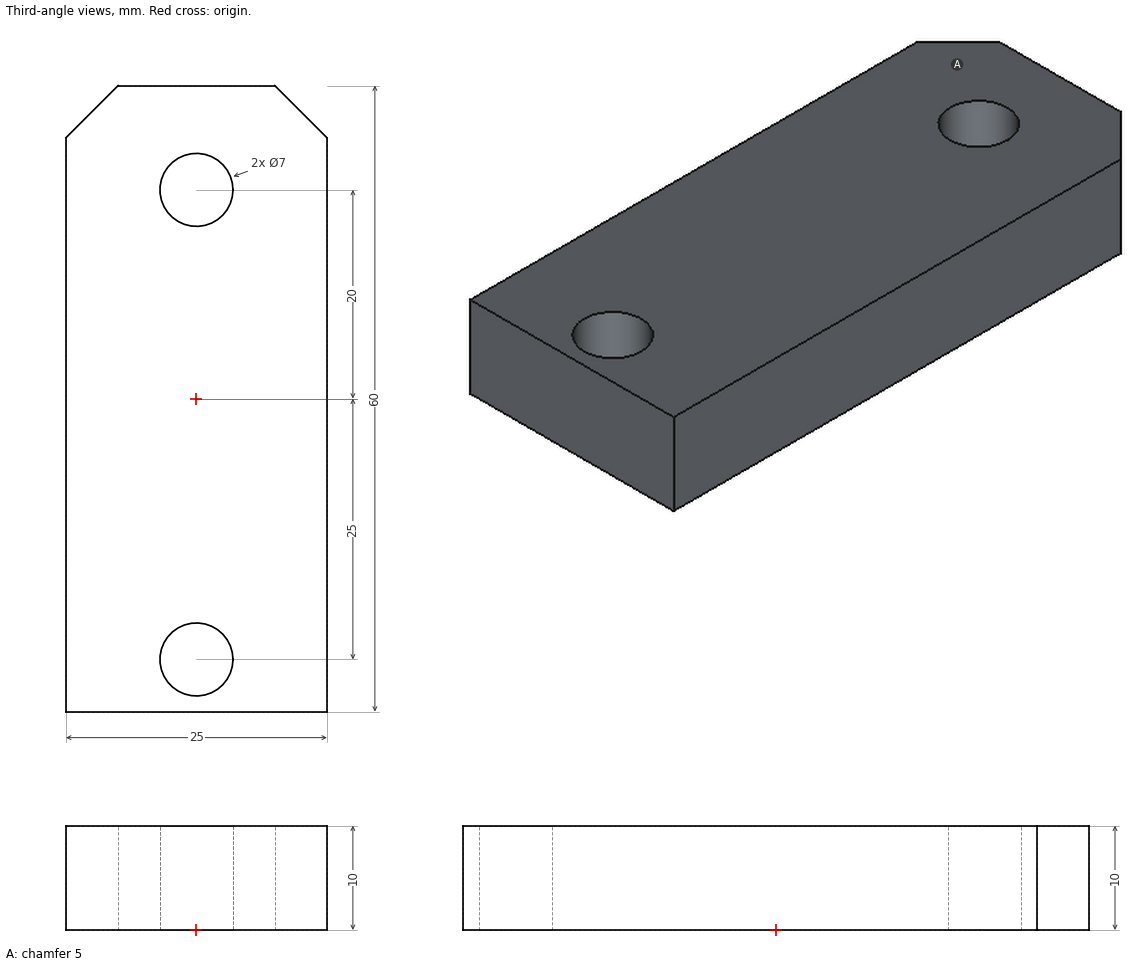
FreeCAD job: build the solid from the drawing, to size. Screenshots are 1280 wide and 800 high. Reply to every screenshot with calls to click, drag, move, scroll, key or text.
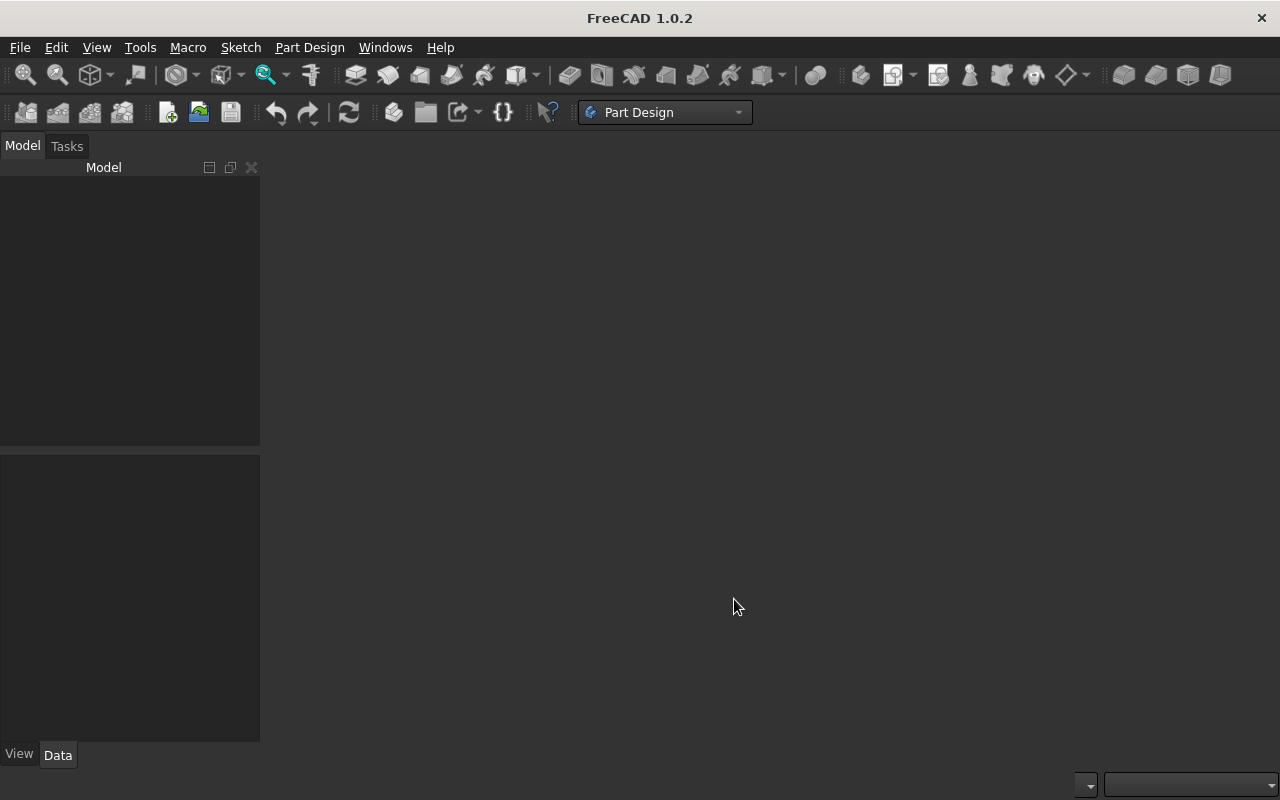
click(168, 112)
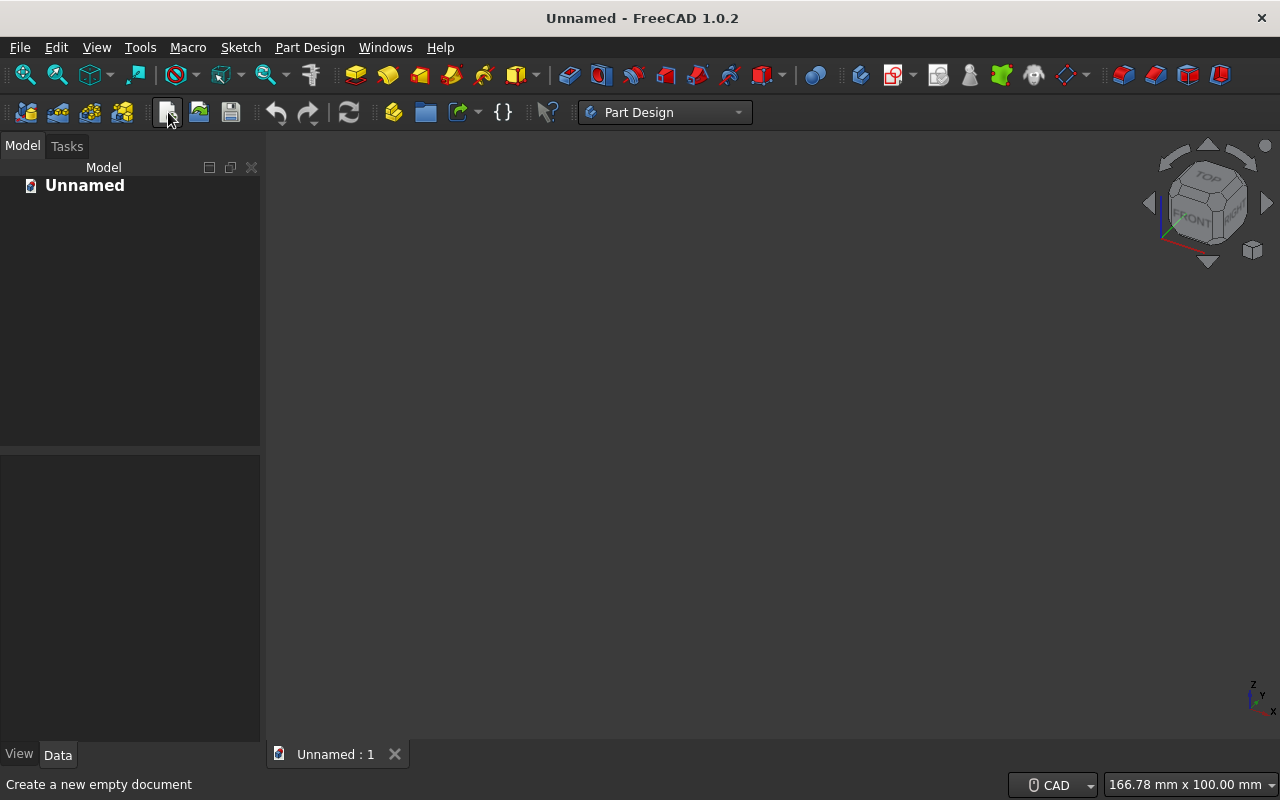
click(894, 76)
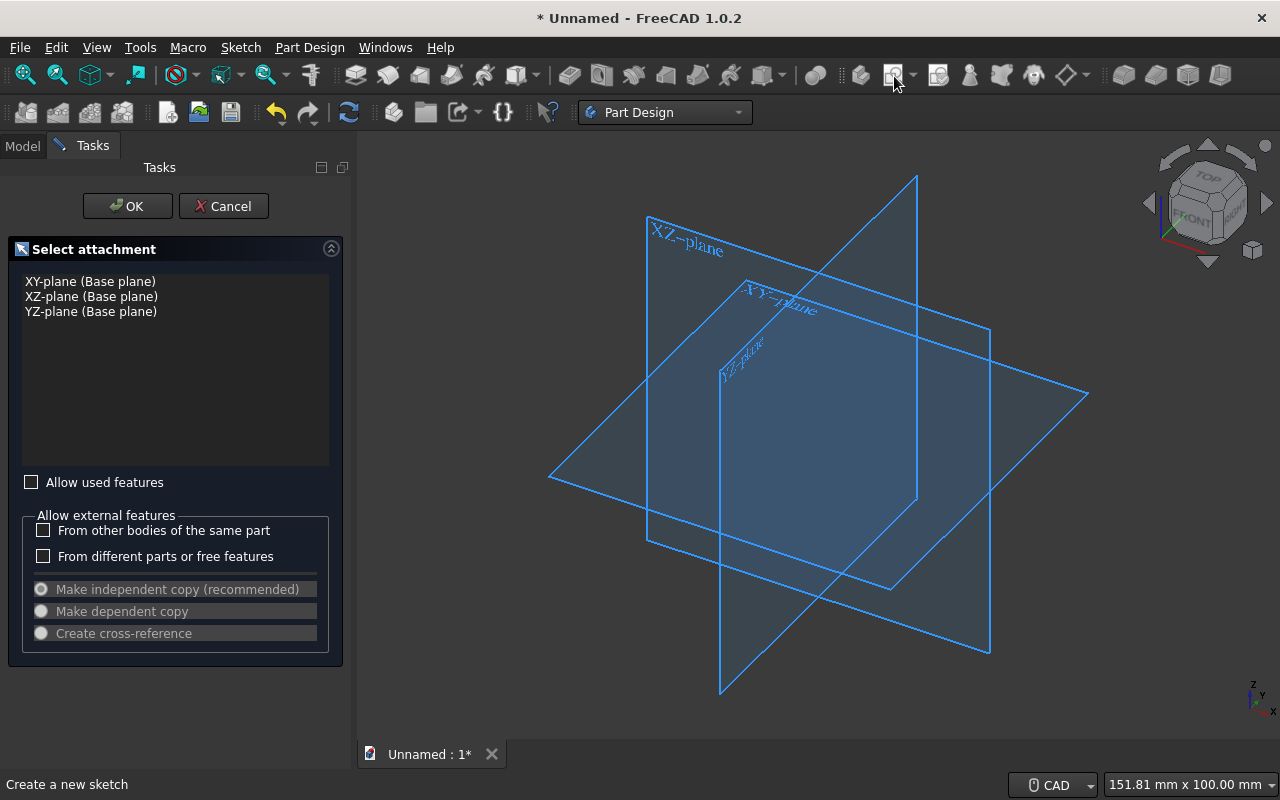
click(82, 282)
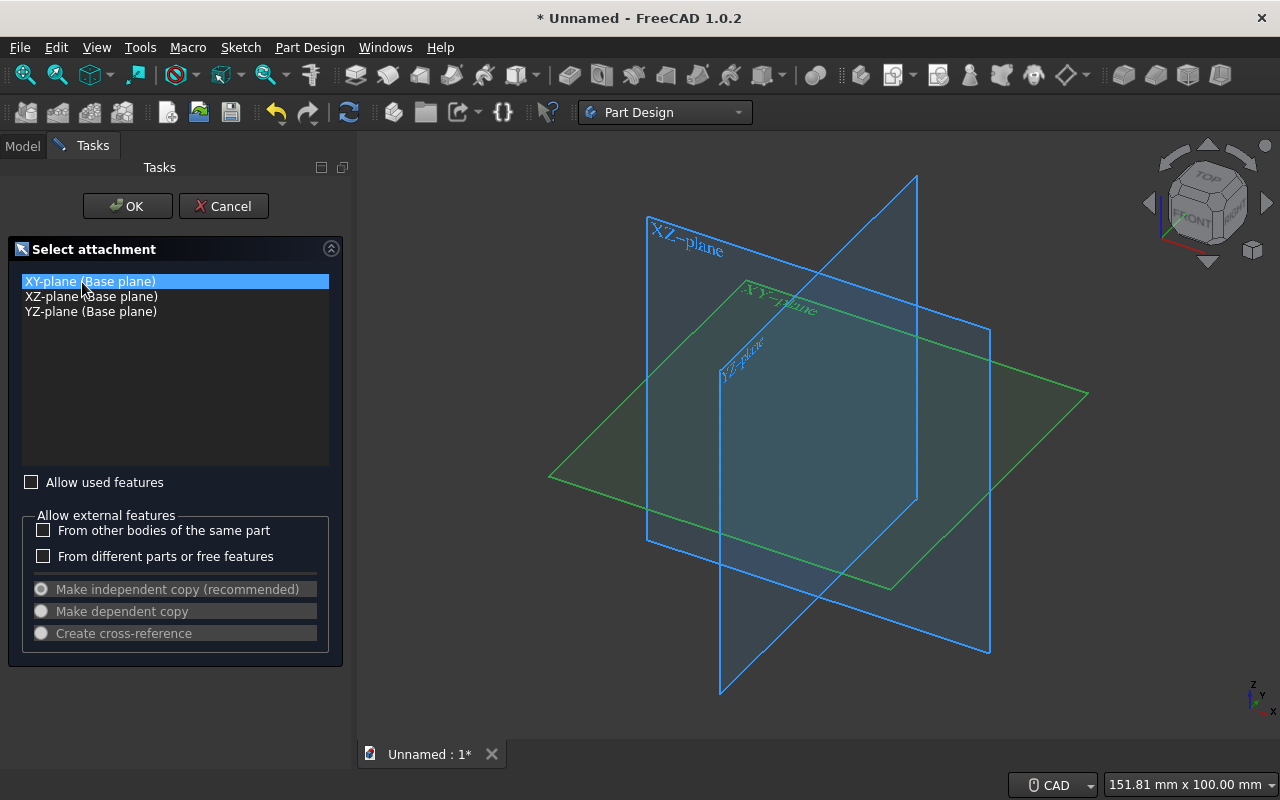
click(128, 206)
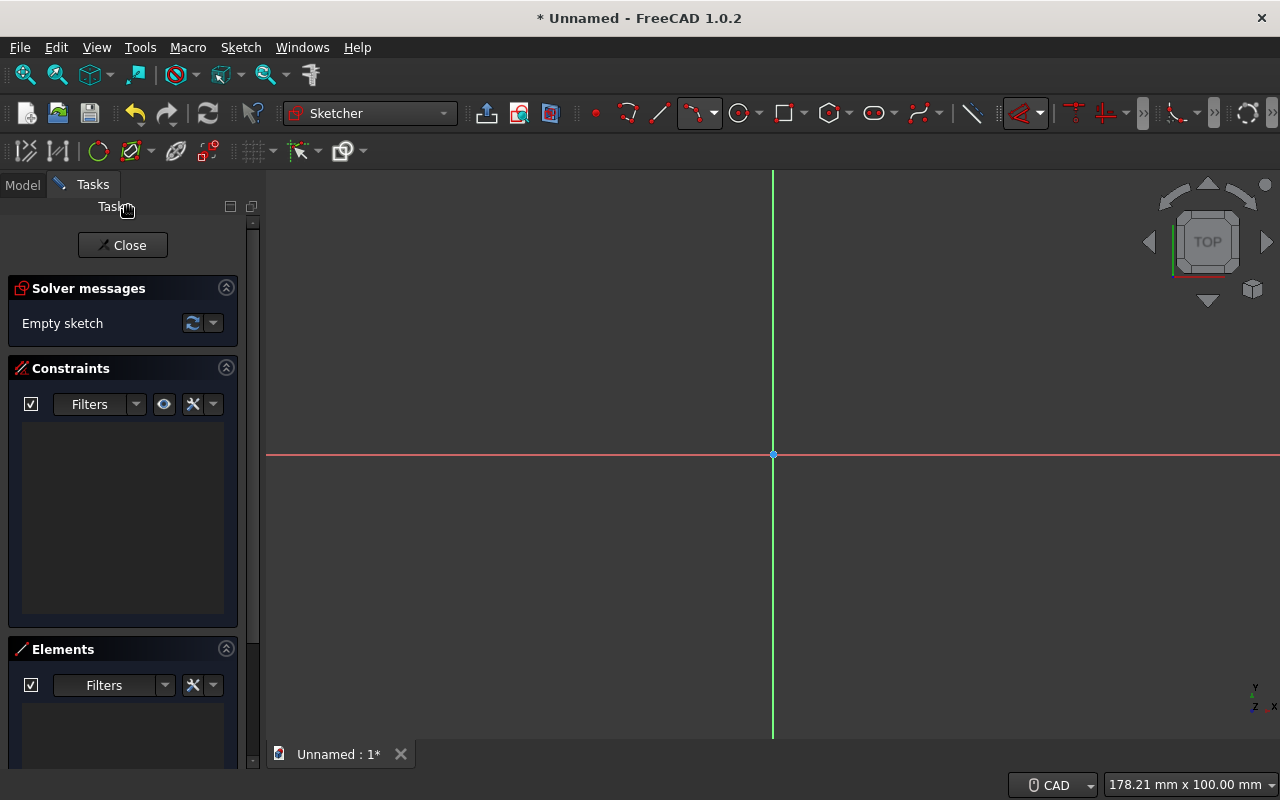
click(806, 114)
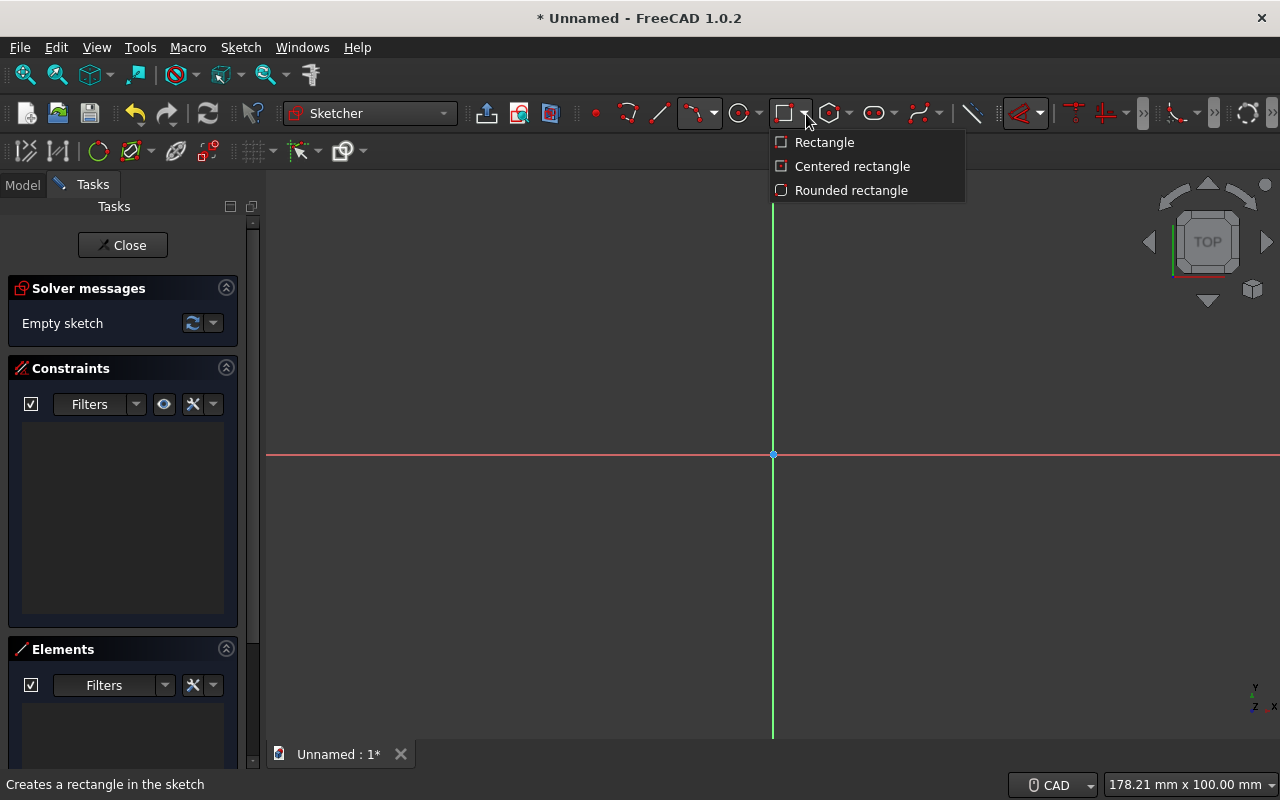
click(868, 166)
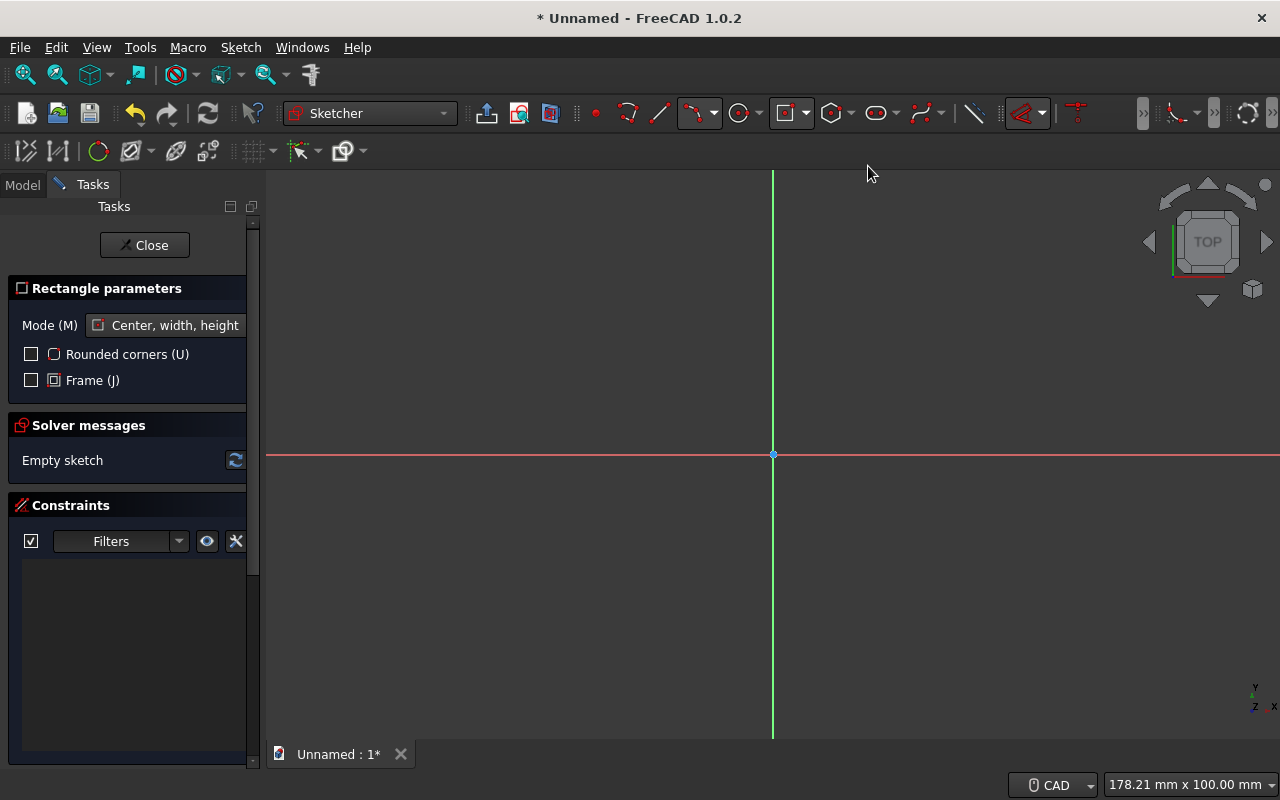
click(773, 454)
click(844, 284)
key(Escape)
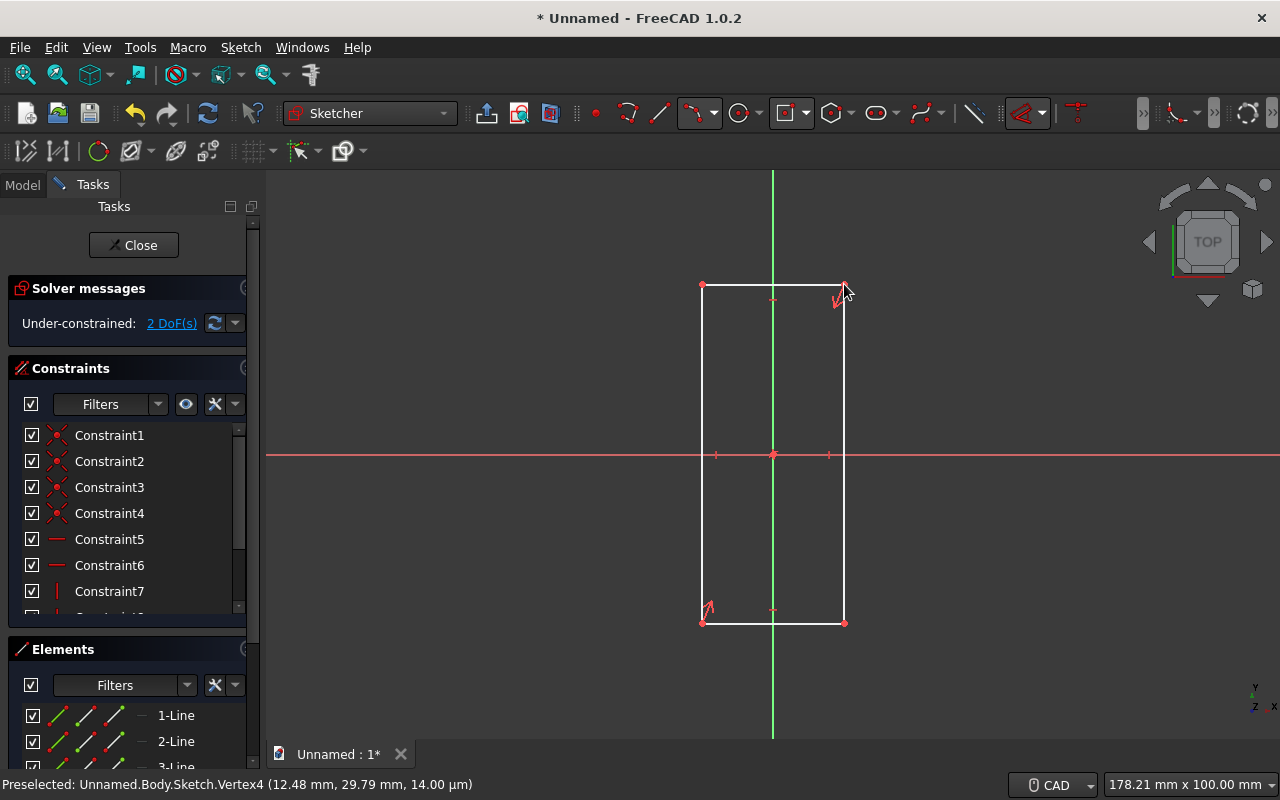
click(1022, 114)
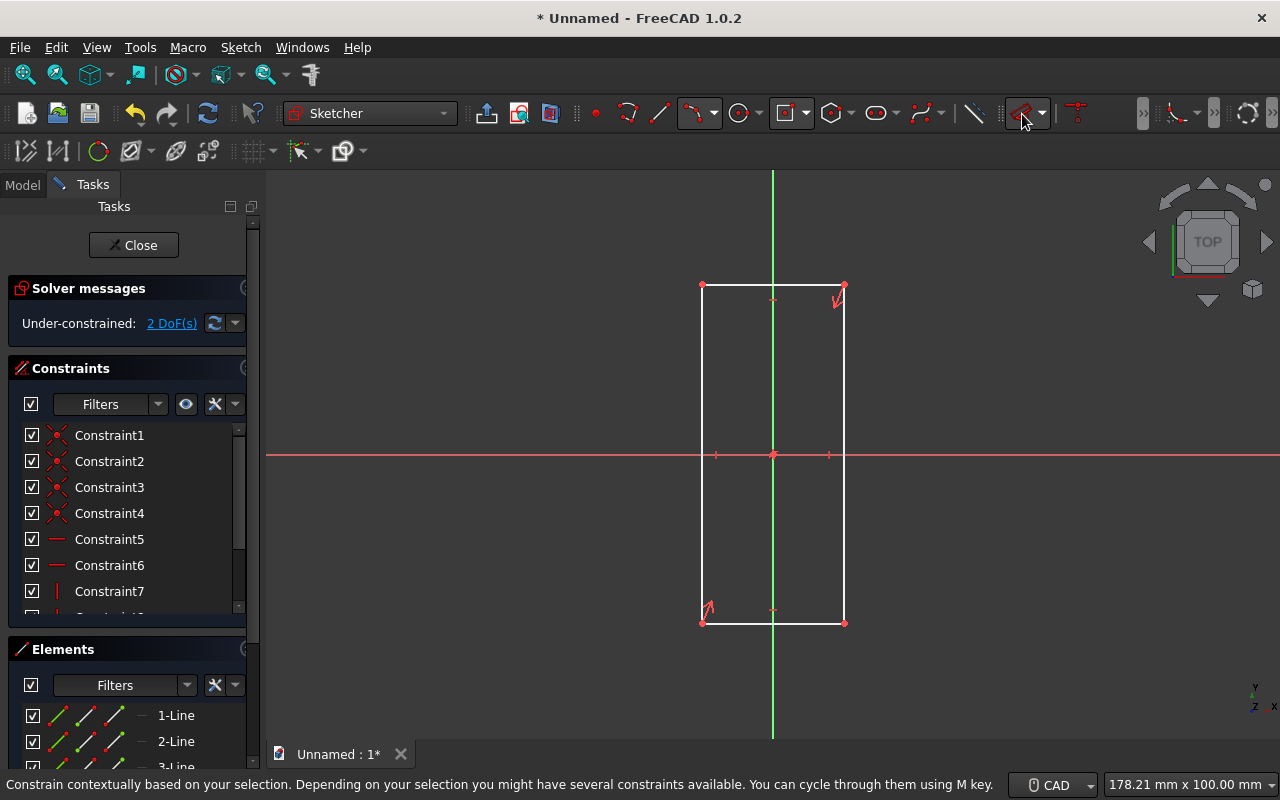
click(745, 624)
click(740, 658)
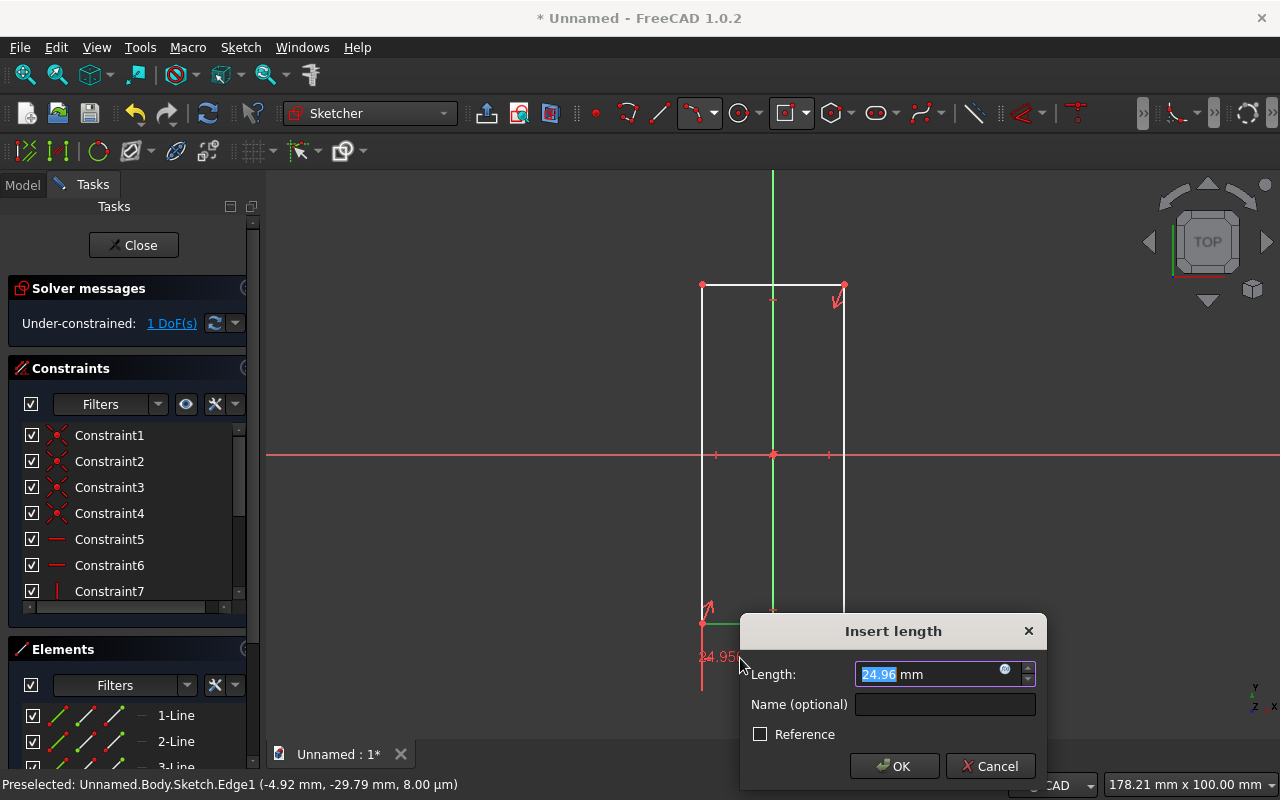
text(25)
key(Return)